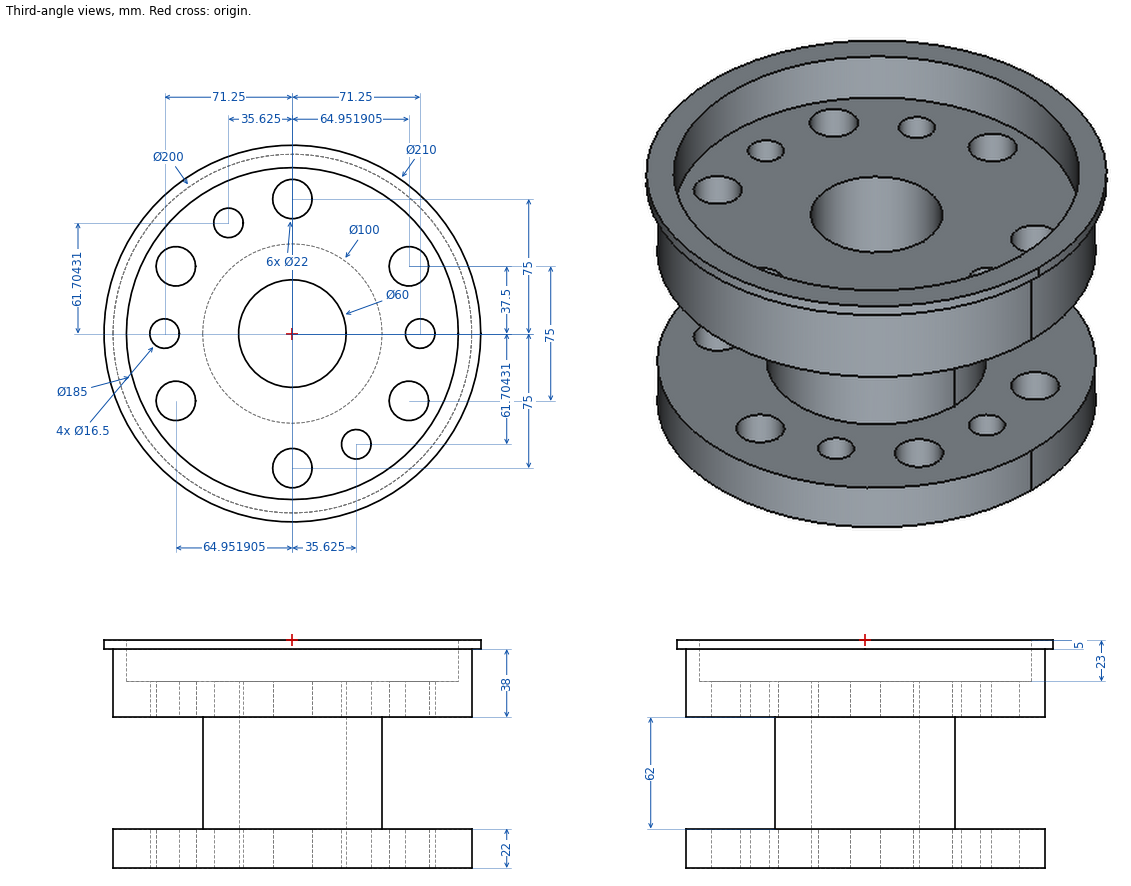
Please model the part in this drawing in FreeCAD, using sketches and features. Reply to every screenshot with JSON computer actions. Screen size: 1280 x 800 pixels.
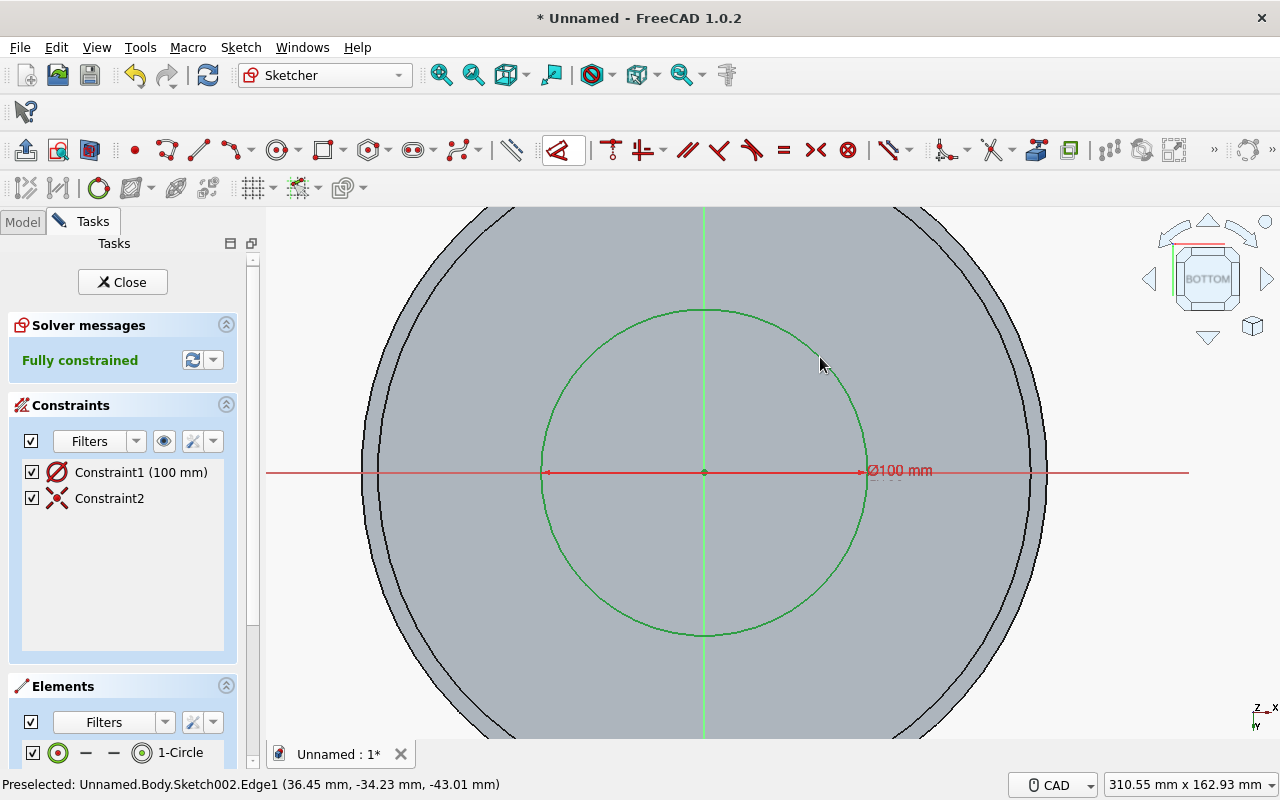
{"action": "left_click", "coordinate": [123, 282]}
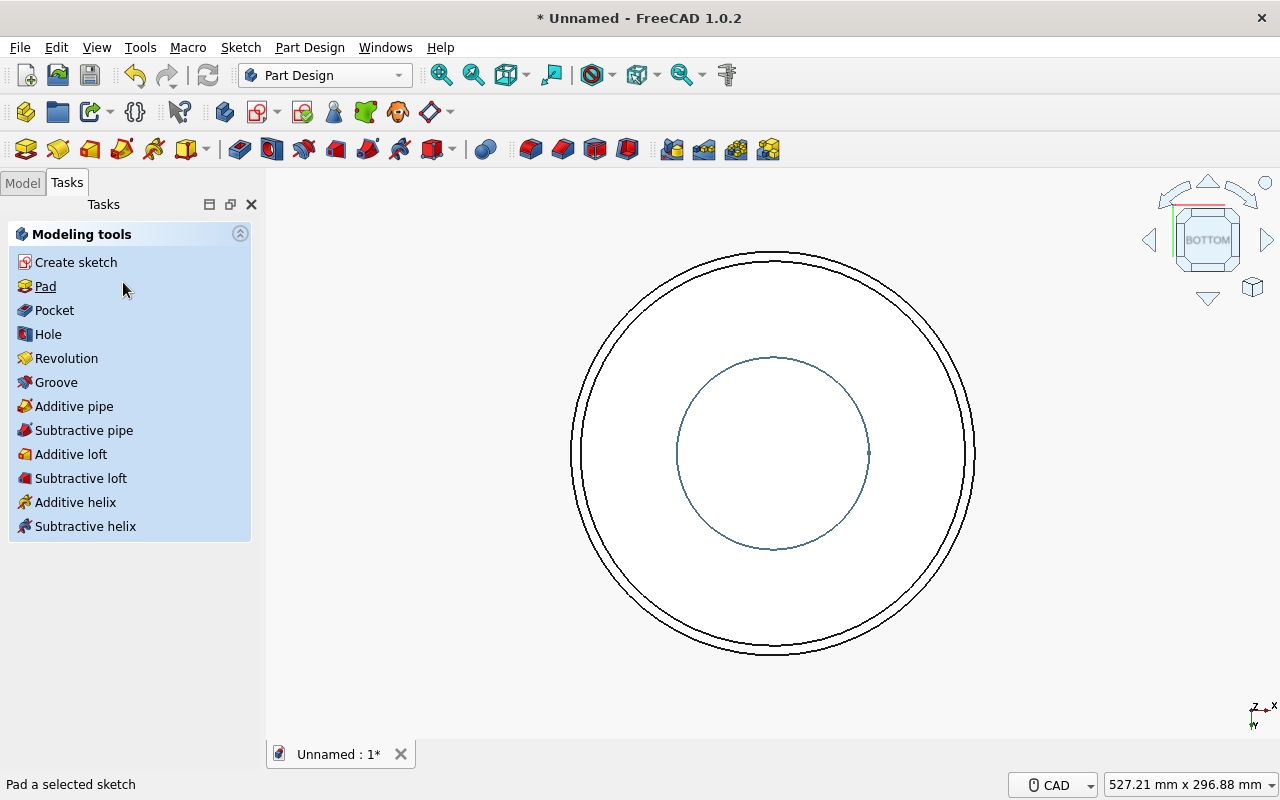
{"action": "left_click", "coordinate": [26, 150]}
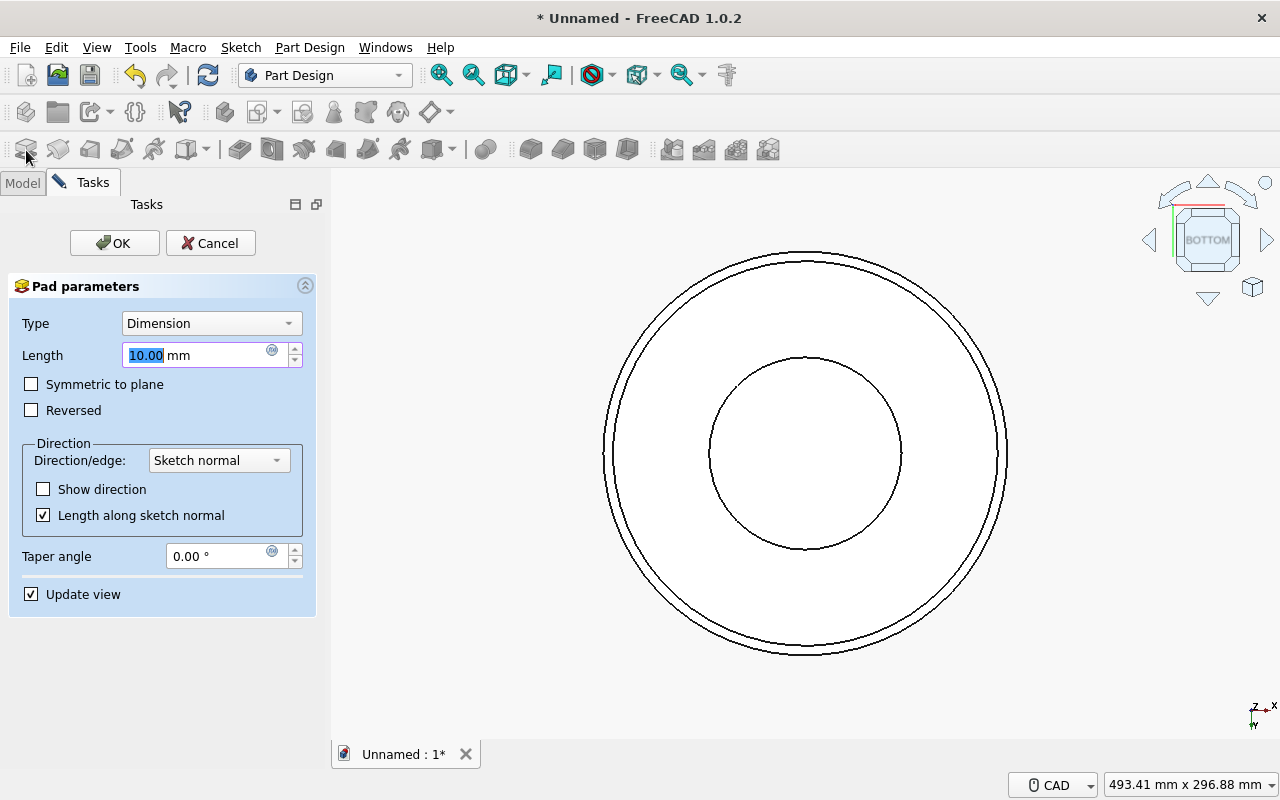
{"action": "type", "text": "62"}
{"action": "key", "text": "Tab"}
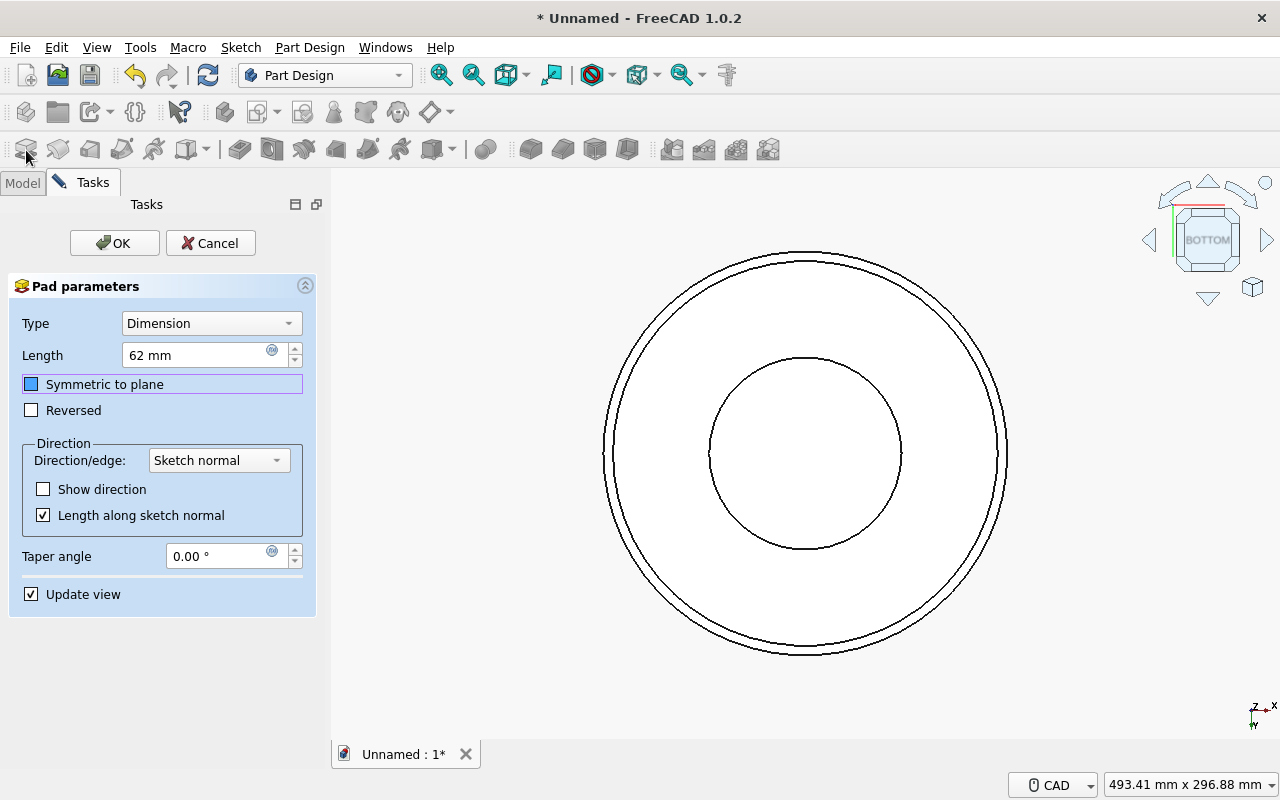
{"action": "left_click", "coordinate": [115, 243]}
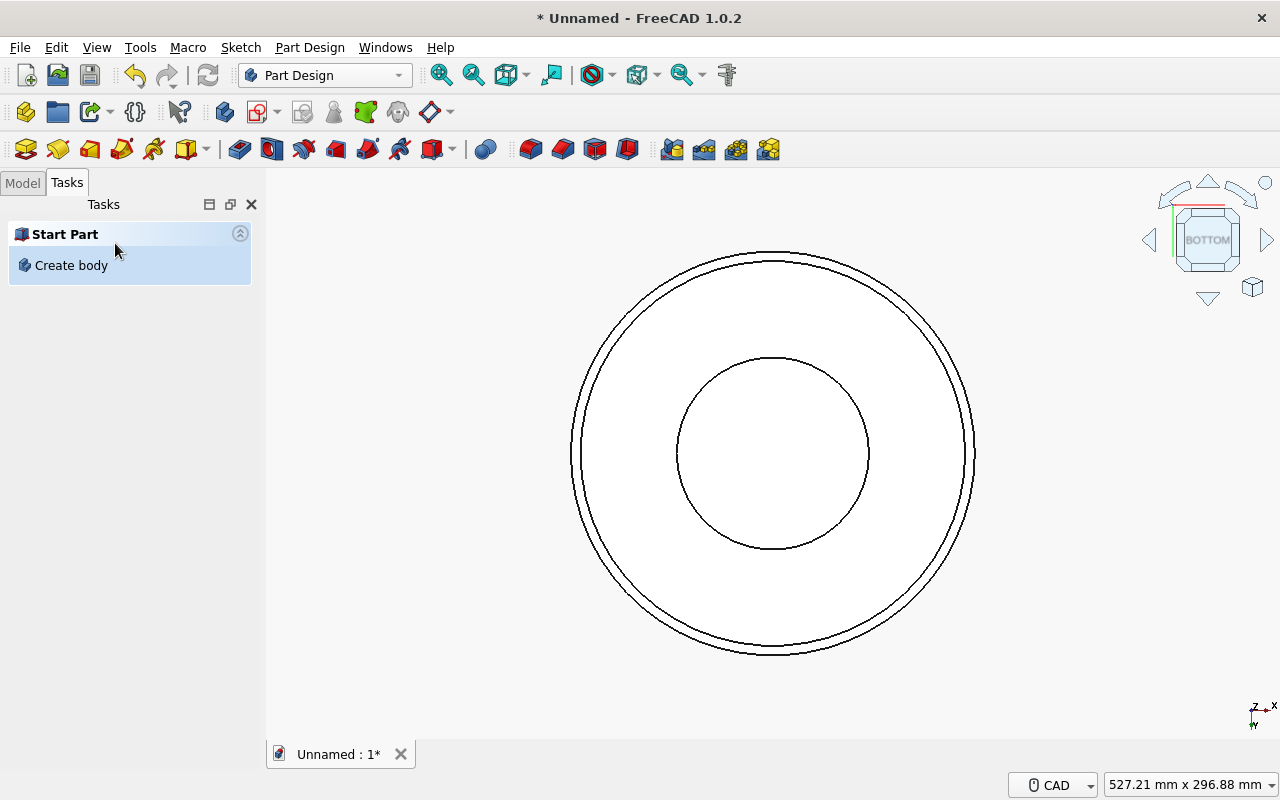
{"action": "left_click", "coordinate": [773, 453]}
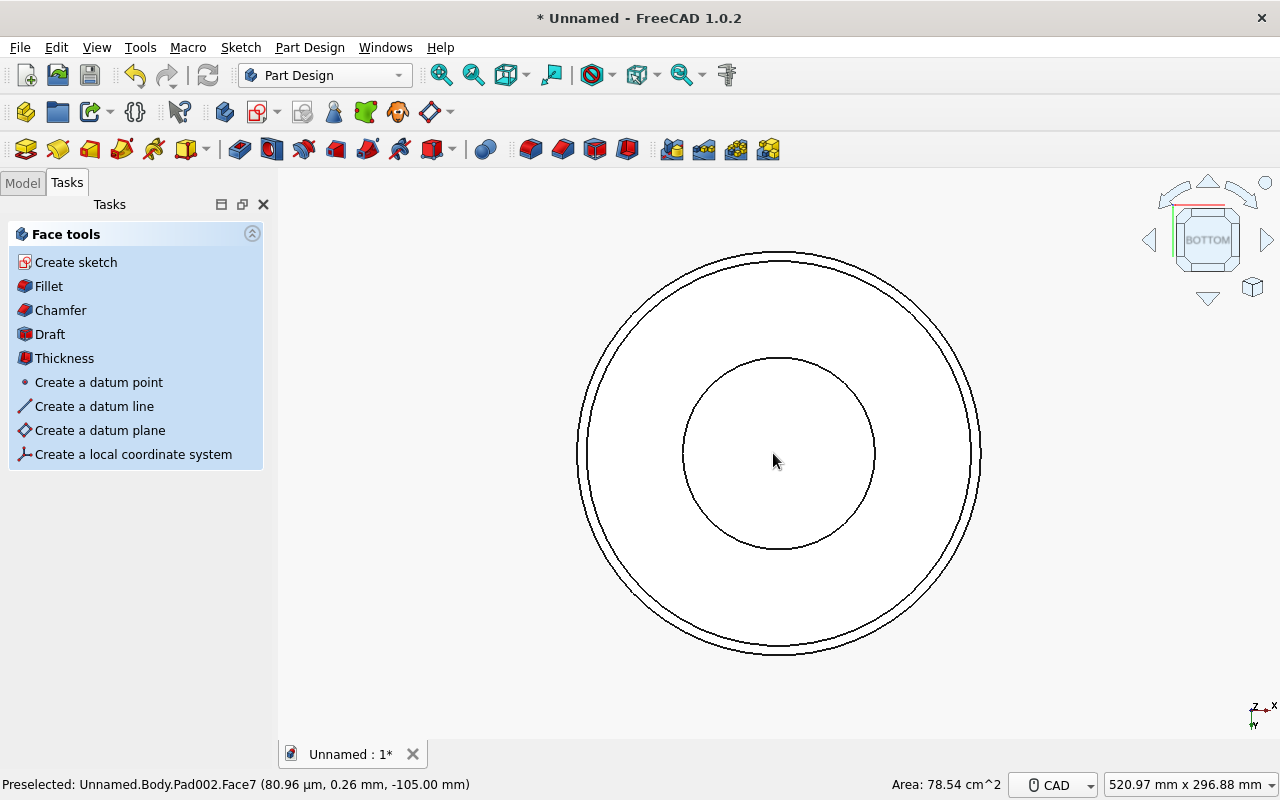
{"action": "left_click", "coordinate": [258, 112]}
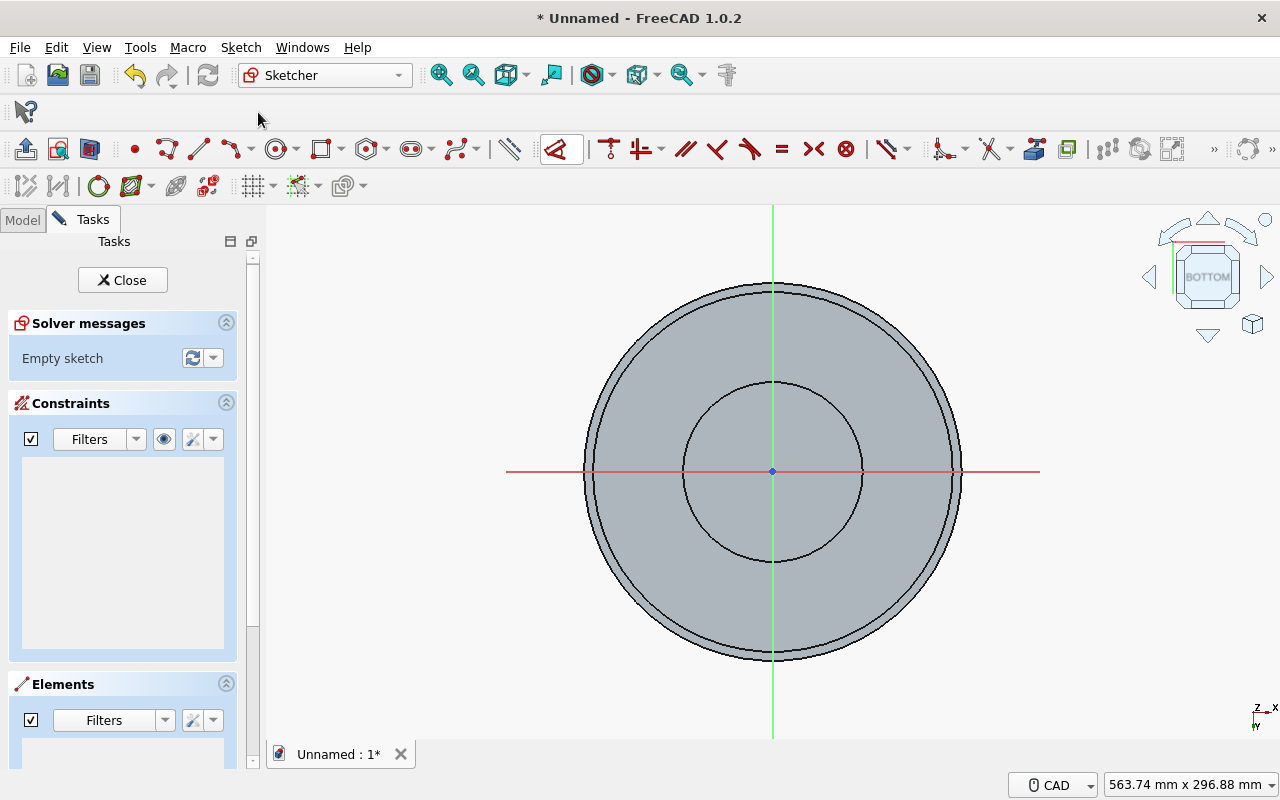
{"action": "left_click", "coordinate": [276, 150]}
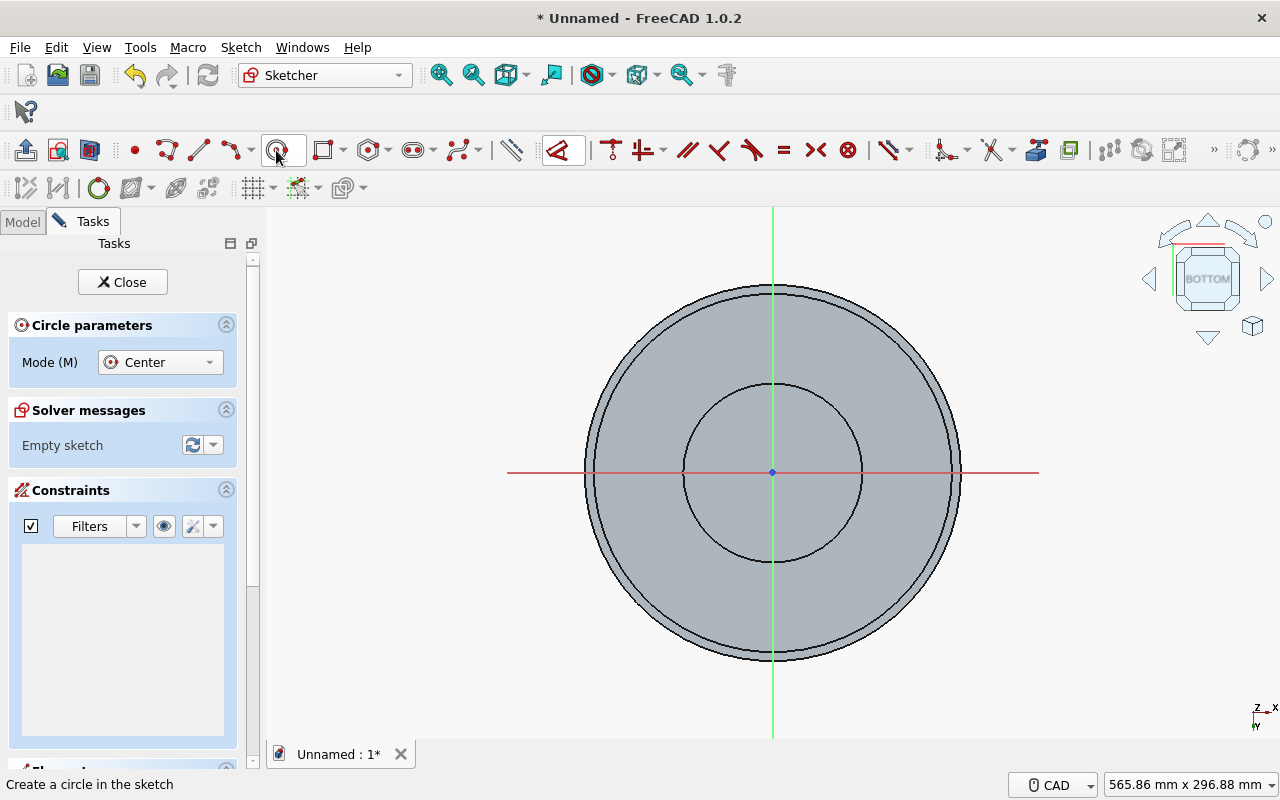
{"action": "left_click", "coordinate": [773, 473]}
{"action": "mouse_move", "coordinate": [900, 346]}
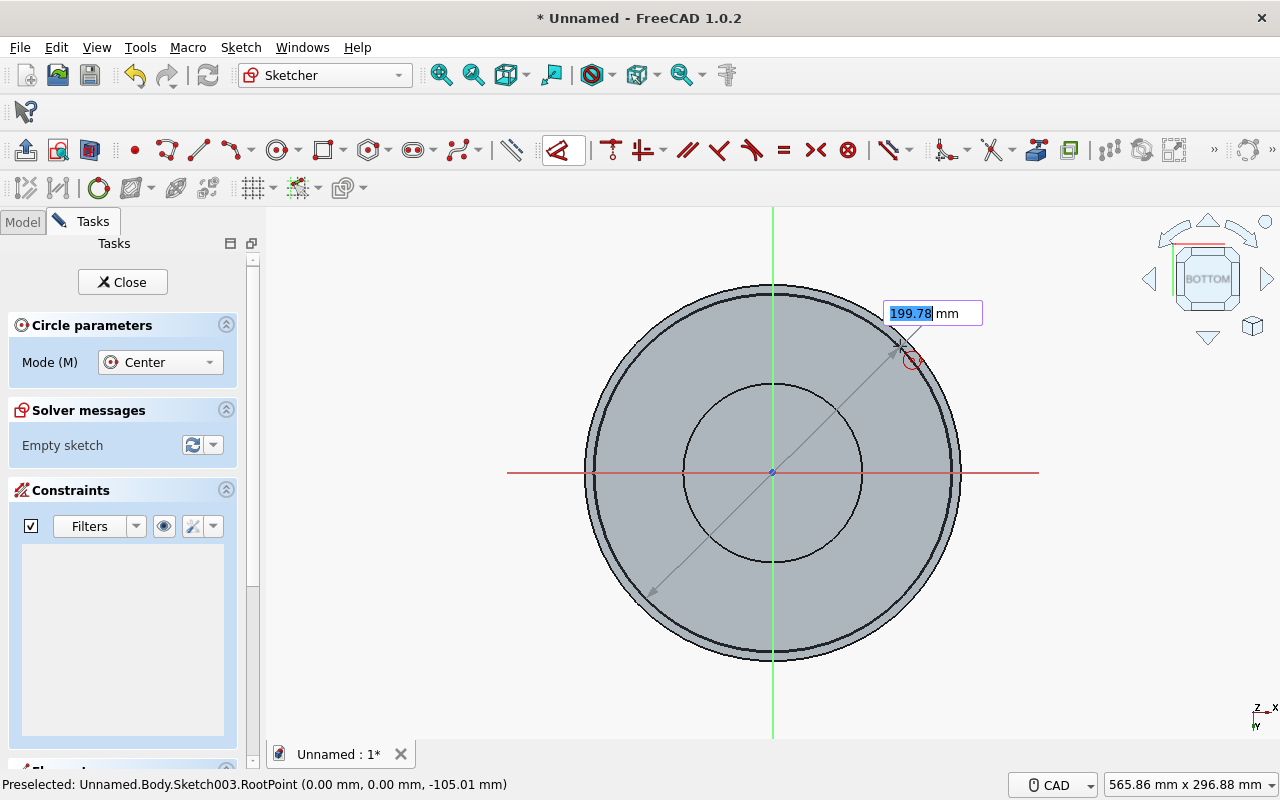
{"action": "type", "text": "200"}
{"action": "key", "text": "Return"}
{"action": "key", "text": "Escape"}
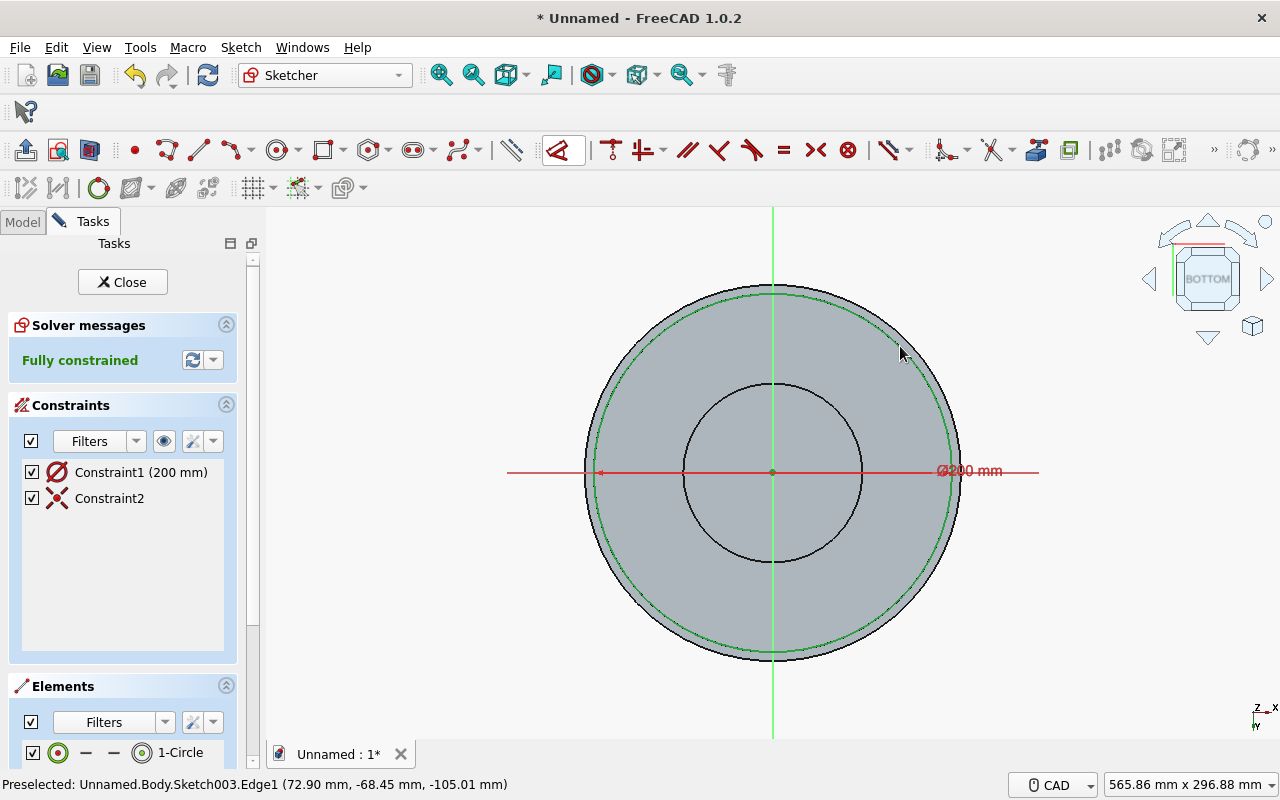
{"action": "left_click", "coordinate": [123, 282]}